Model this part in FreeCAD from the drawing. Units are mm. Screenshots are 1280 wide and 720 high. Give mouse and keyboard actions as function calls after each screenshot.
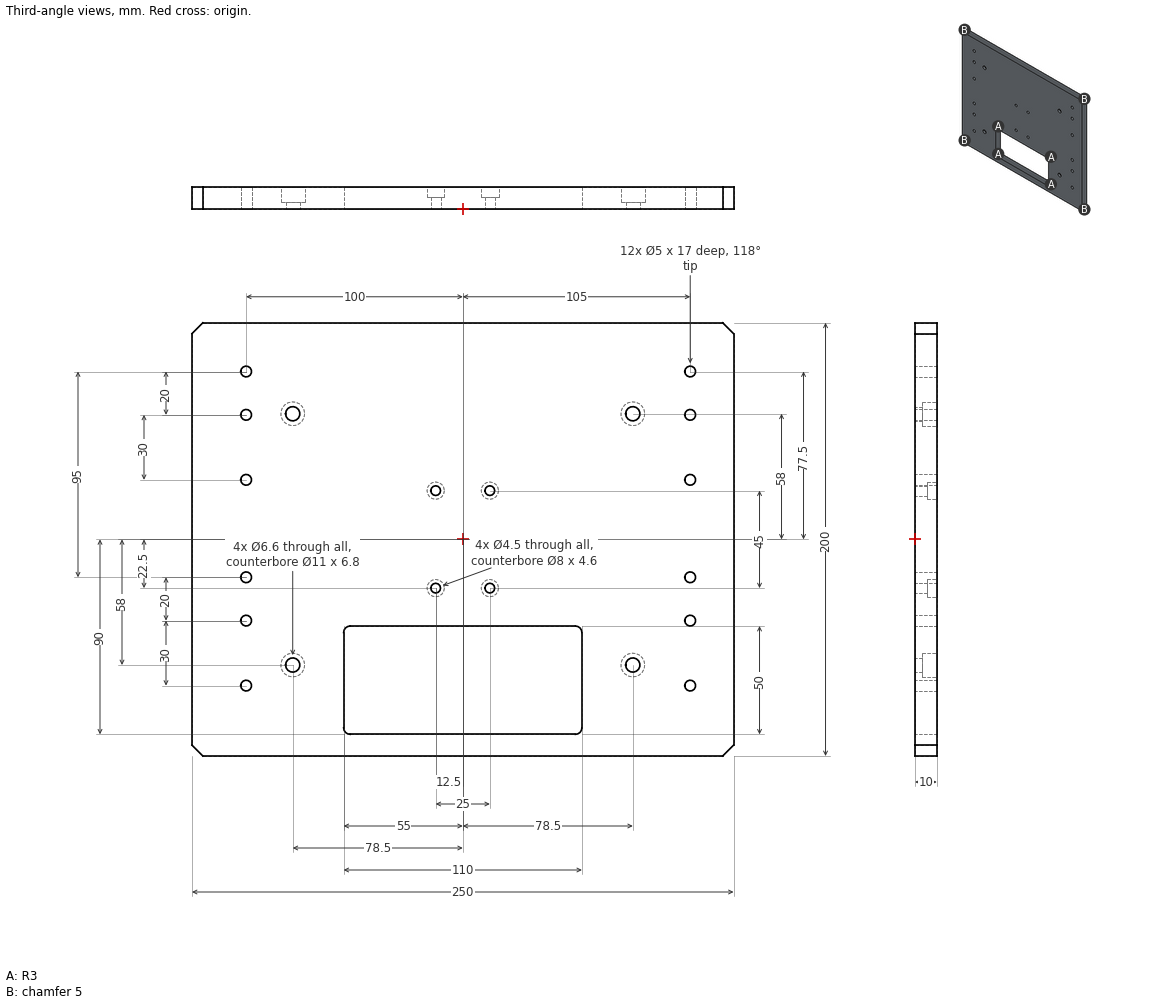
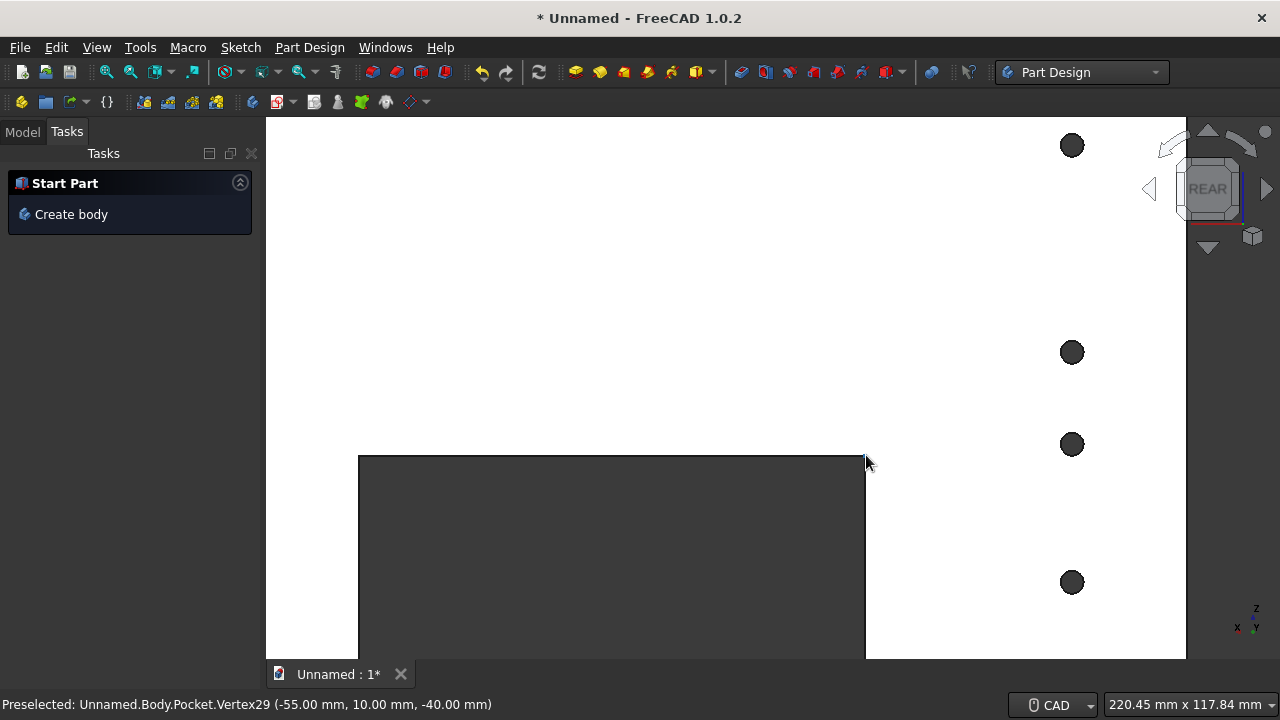
click(108, 72)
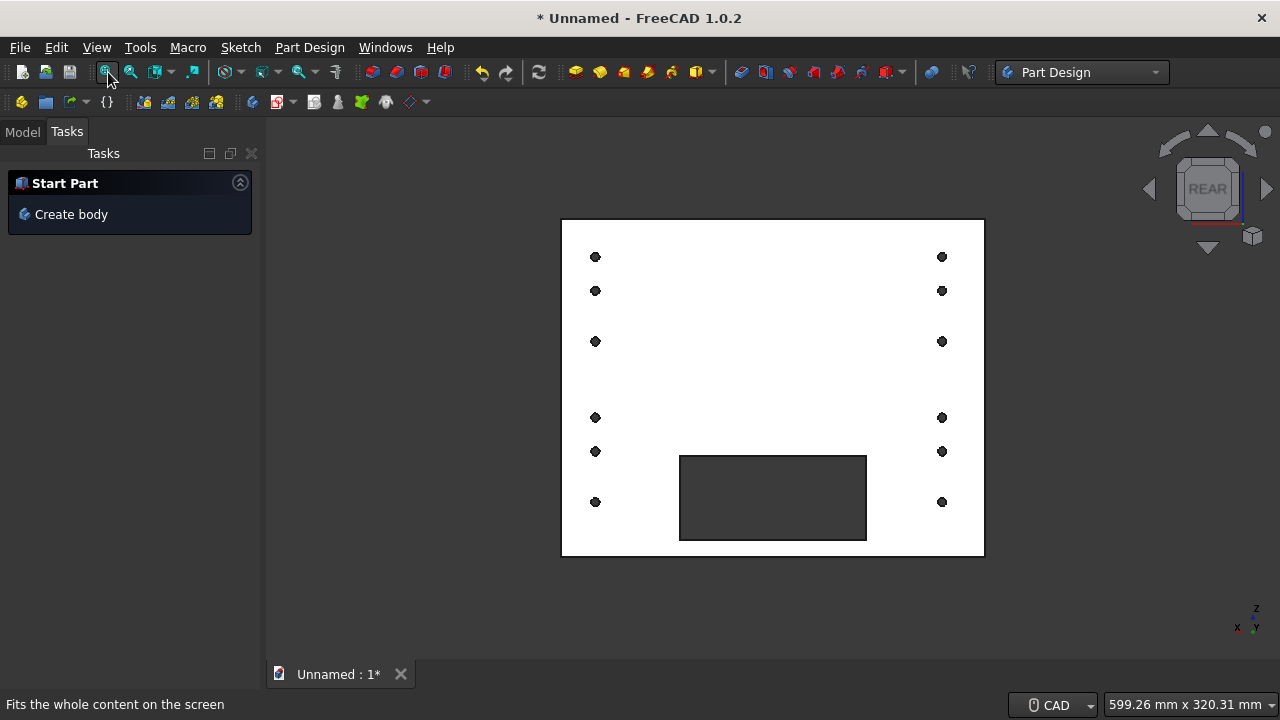
key(0)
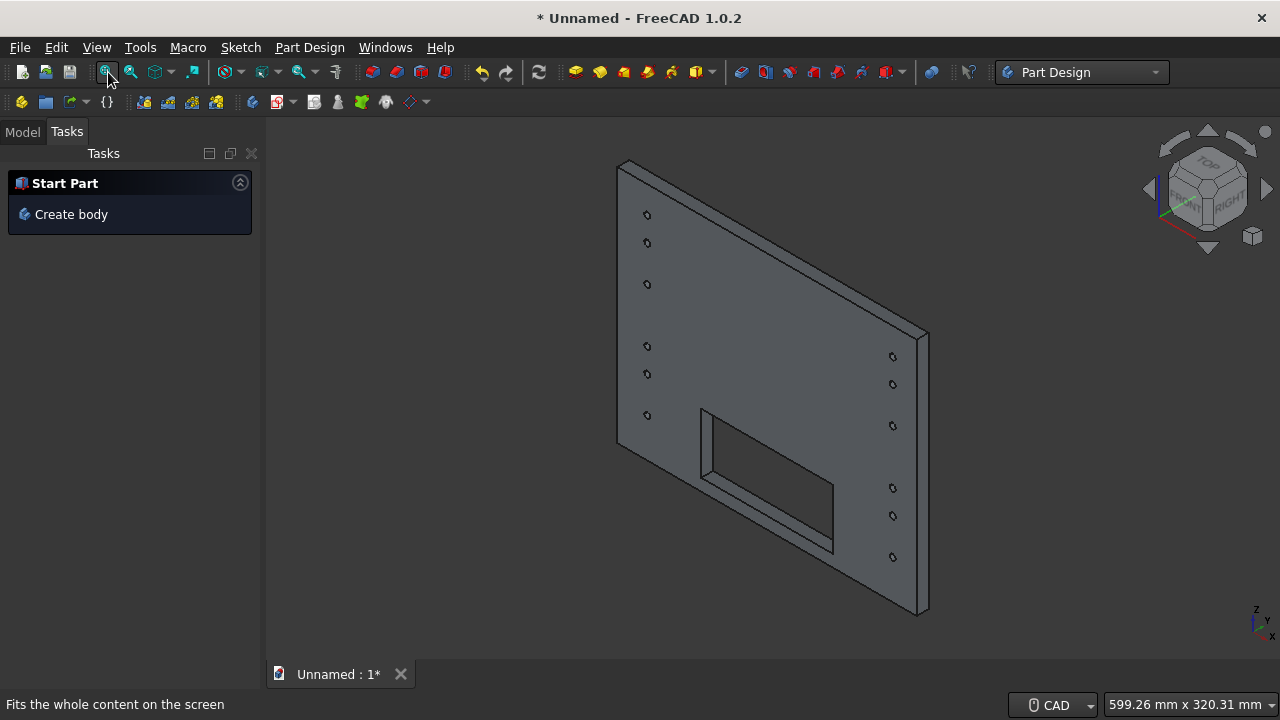
scroll(707, 404, up, 5)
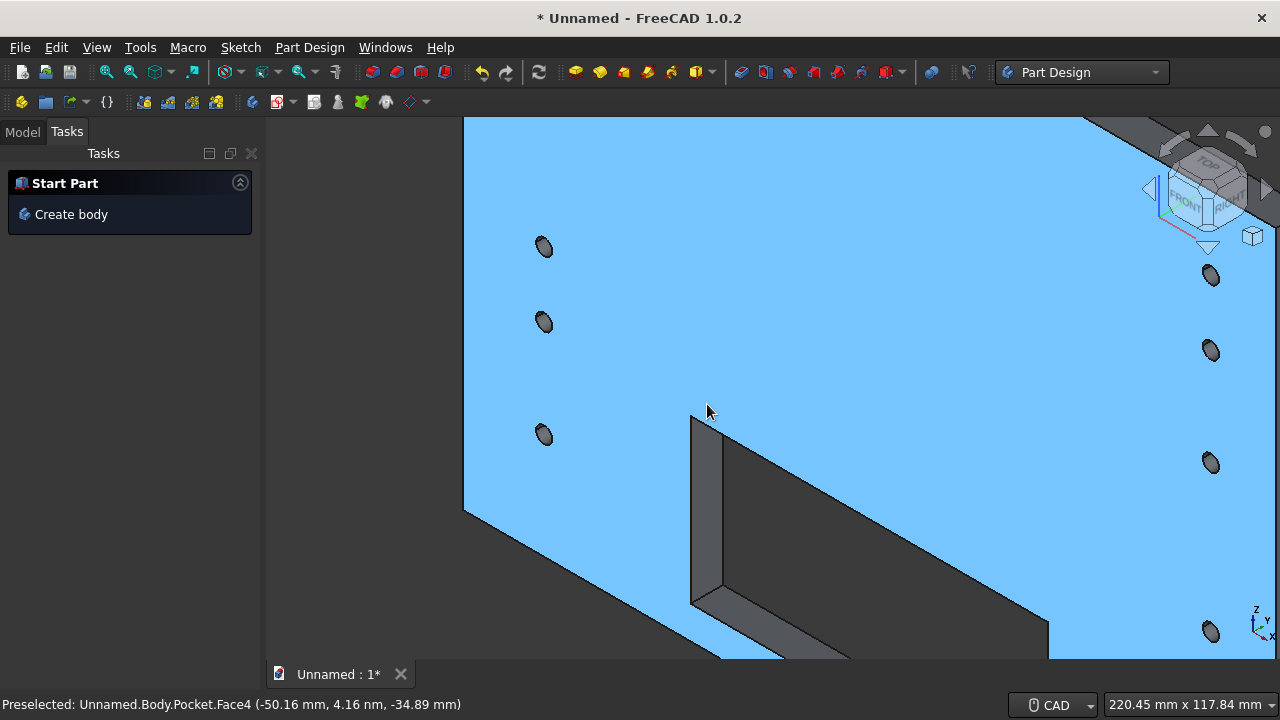
click(108, 72)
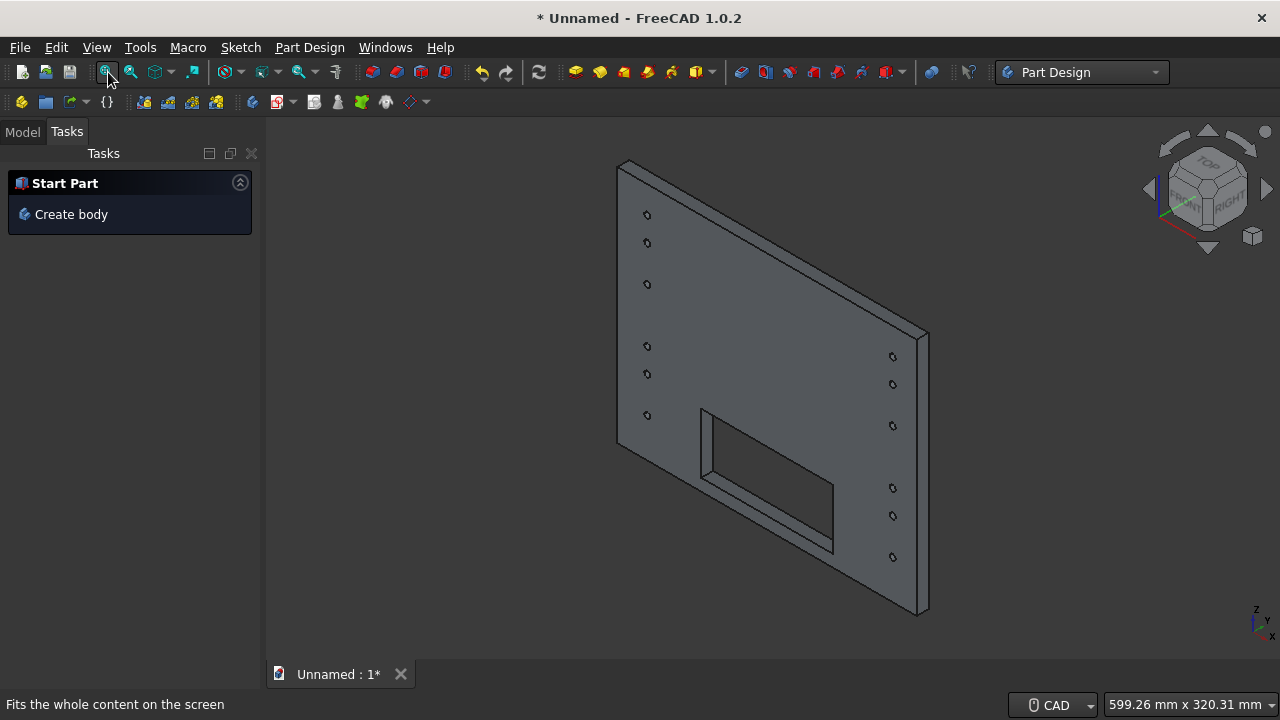
key(2)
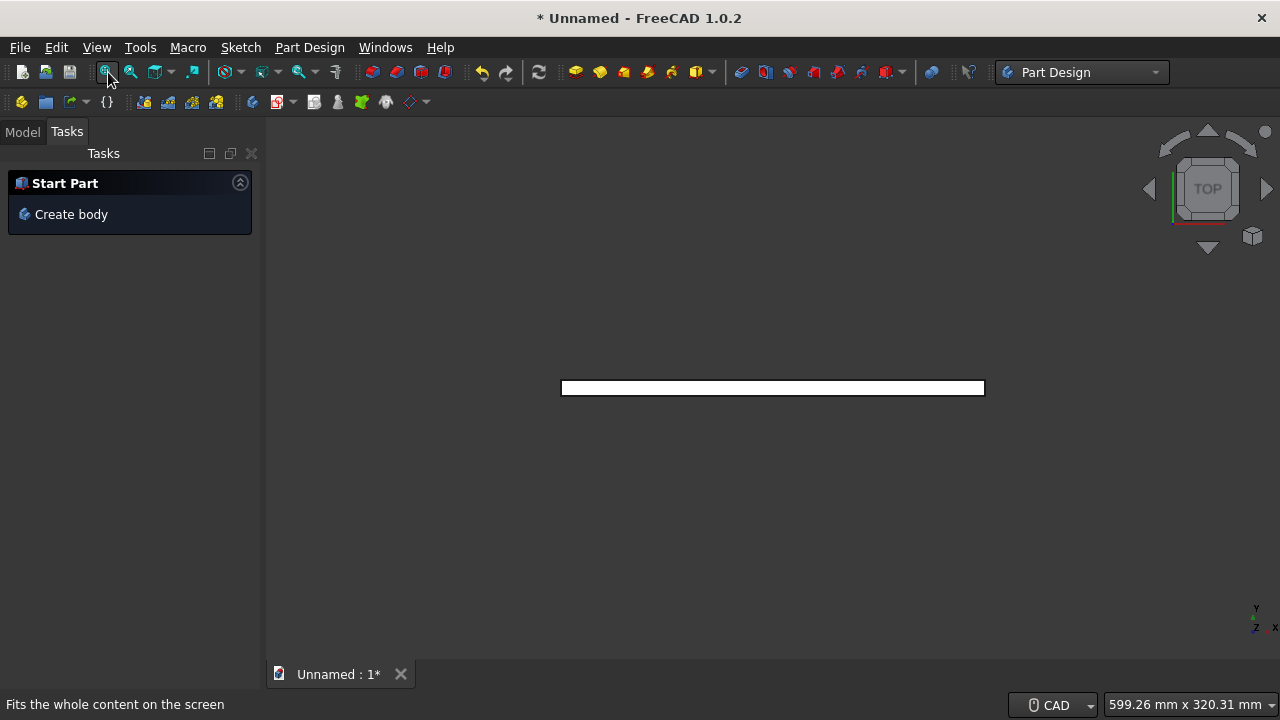
click(108, 72)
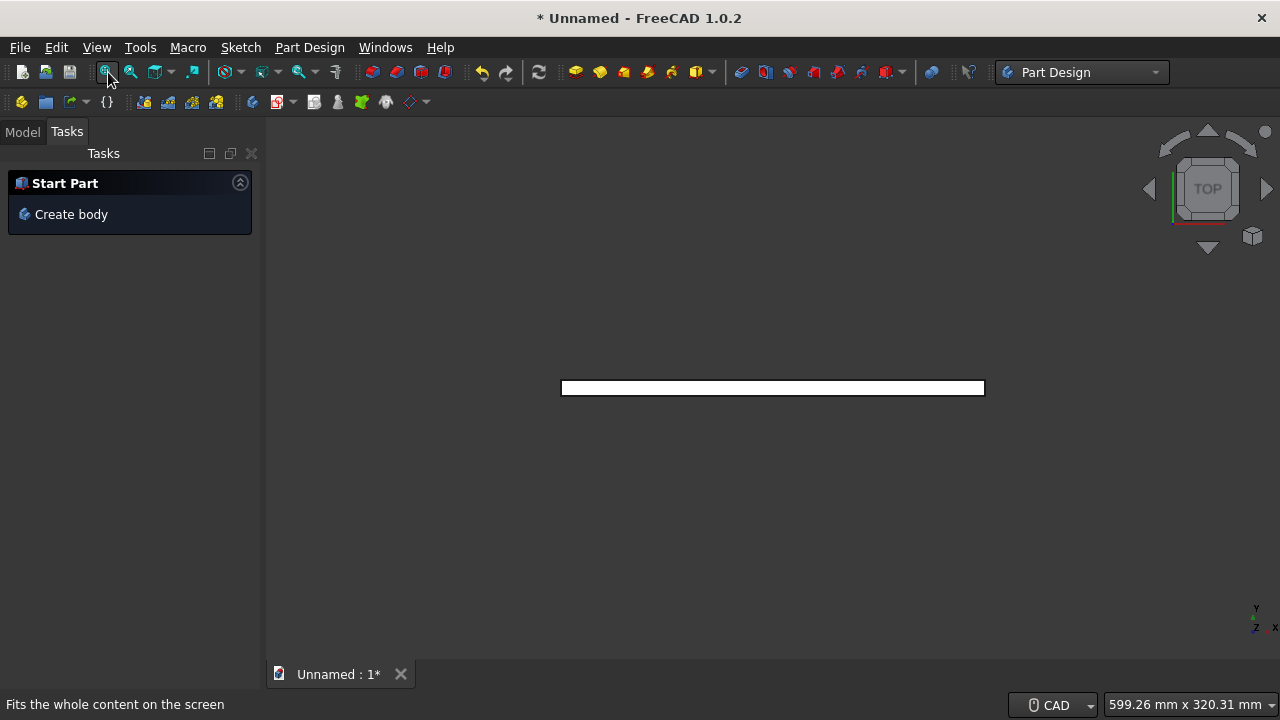
scroll(680, 387, up, 5)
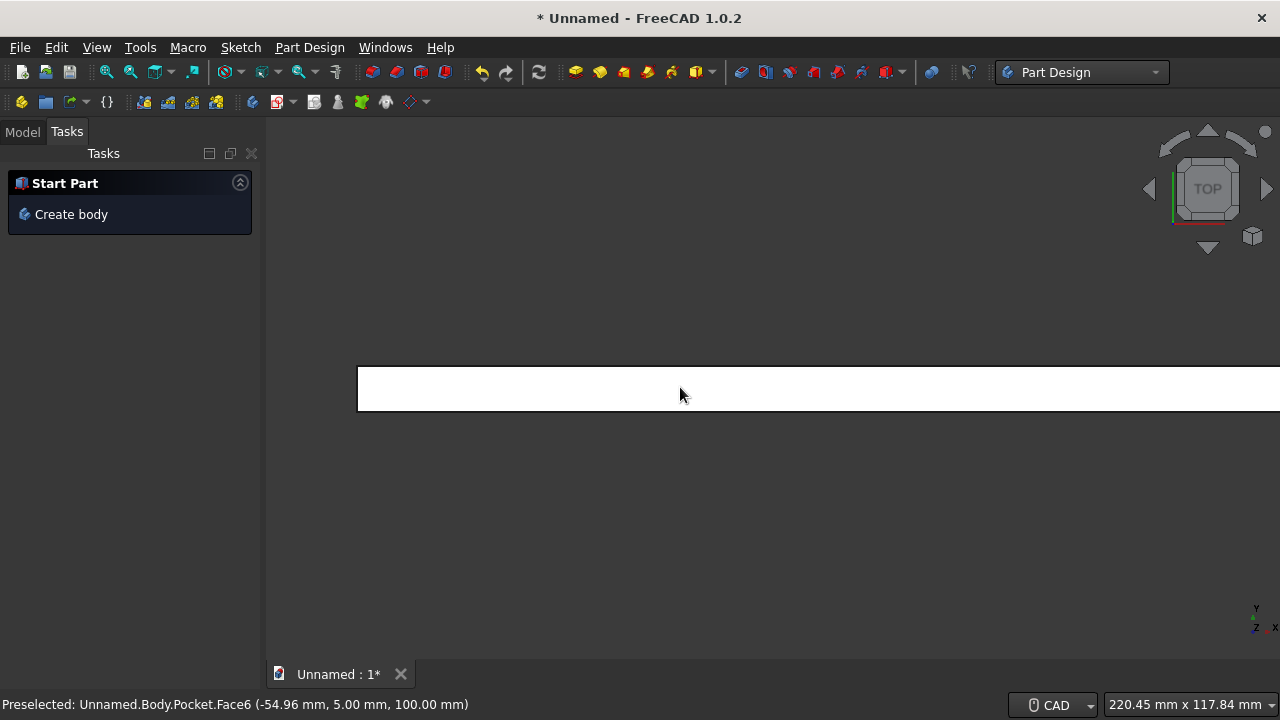
click(108, 72)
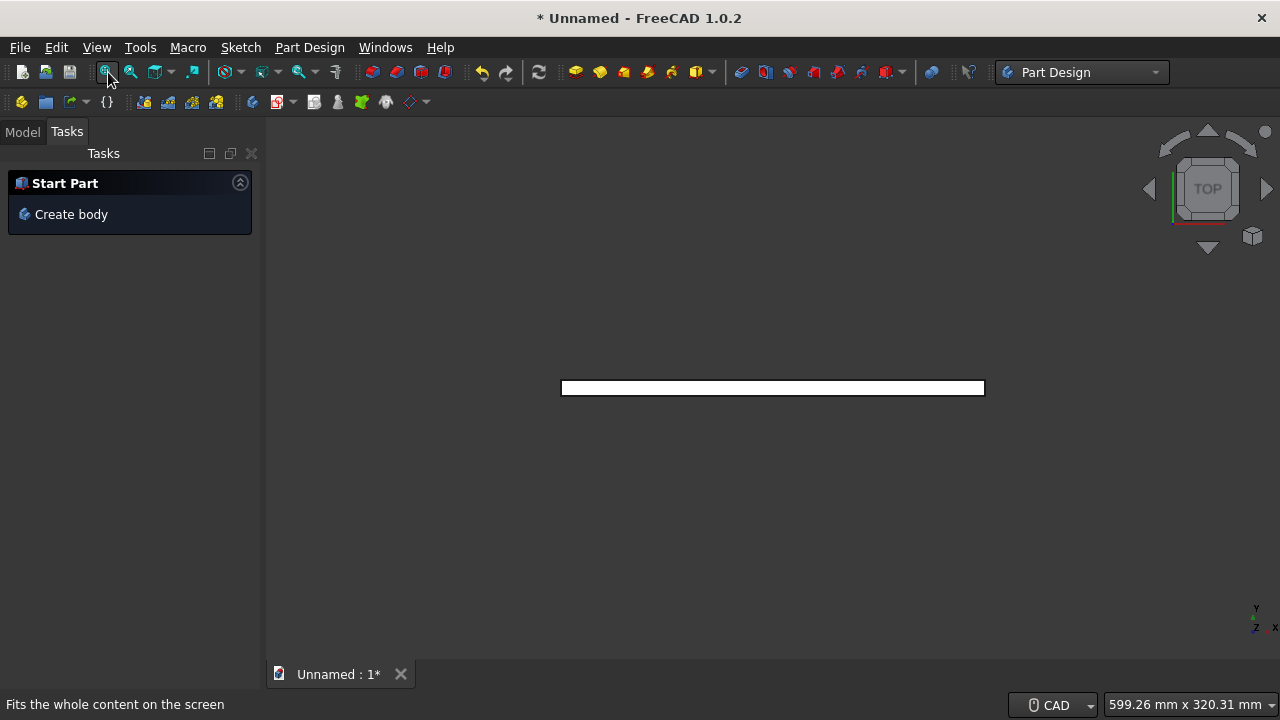
key(1)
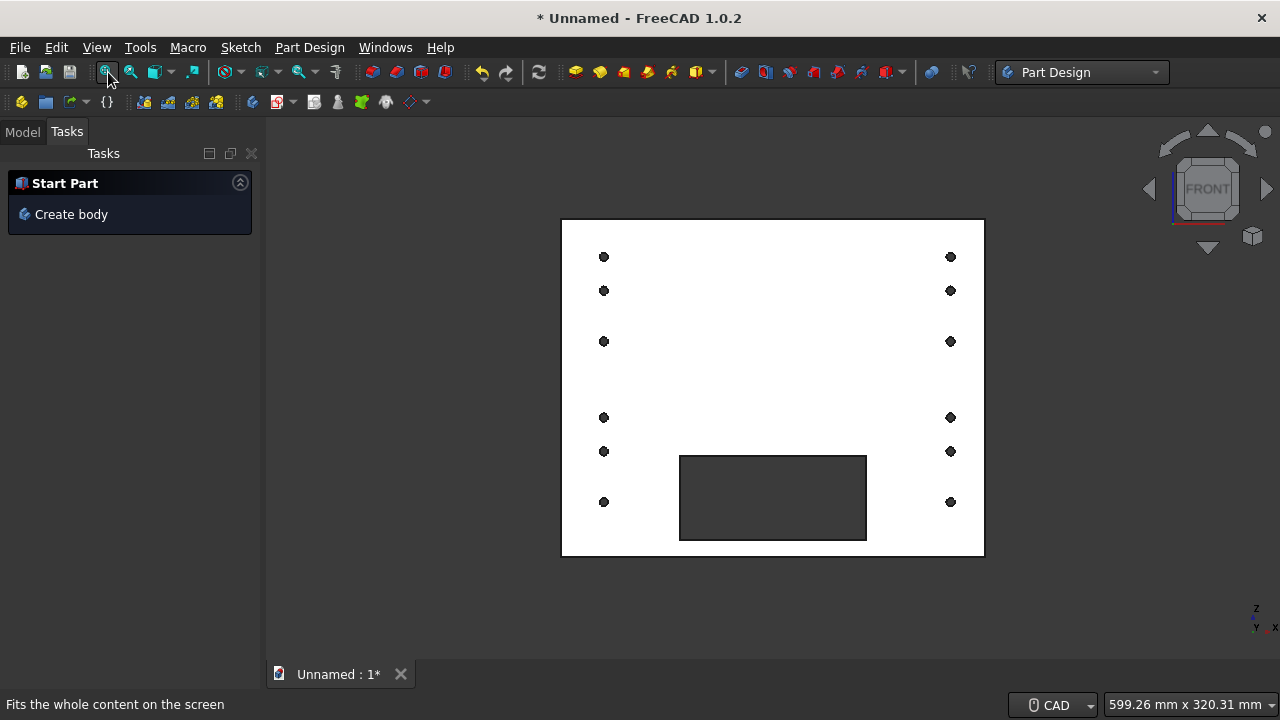
scroll(680, 455, up, 5)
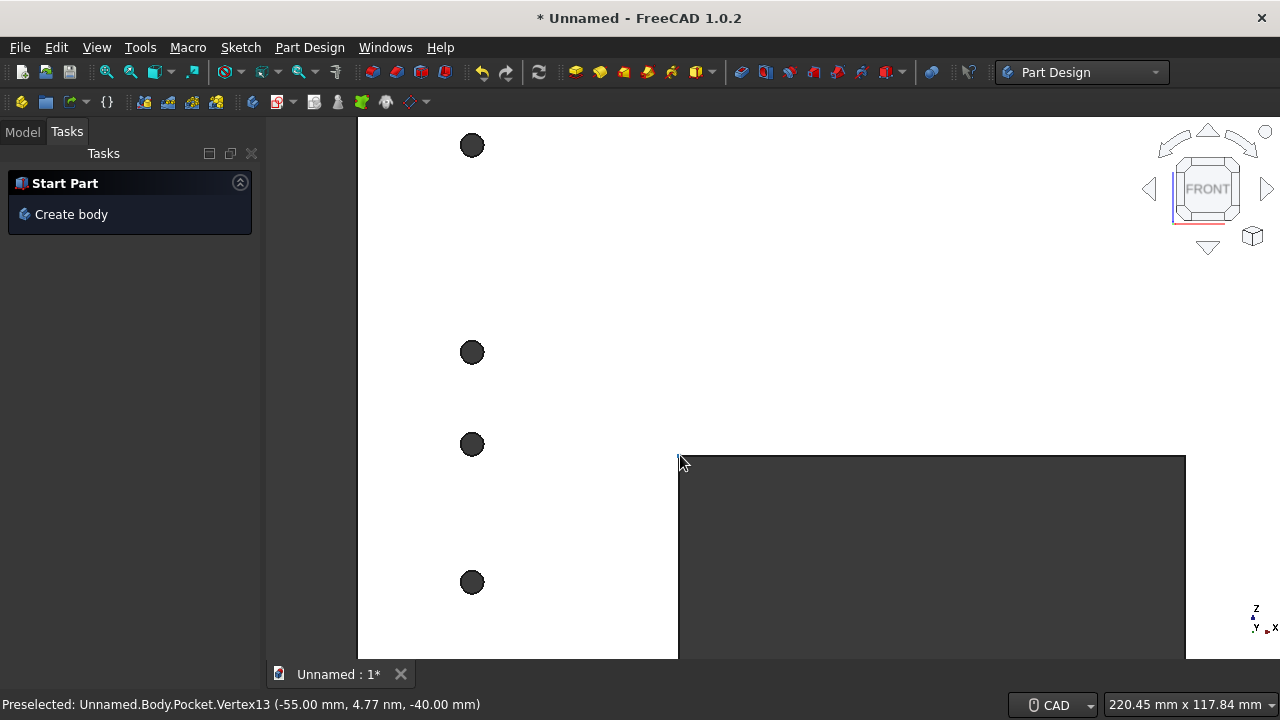
click(108, 72)